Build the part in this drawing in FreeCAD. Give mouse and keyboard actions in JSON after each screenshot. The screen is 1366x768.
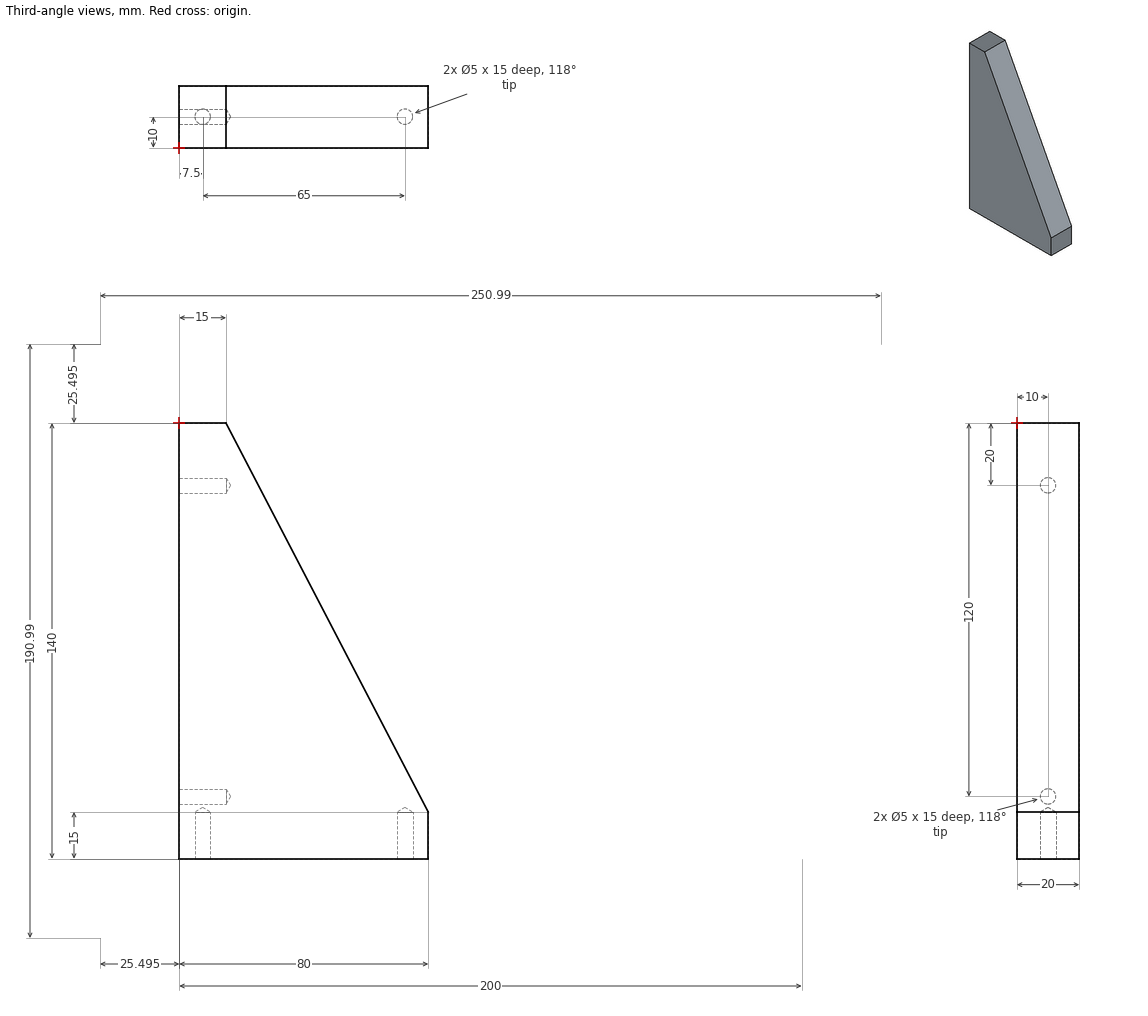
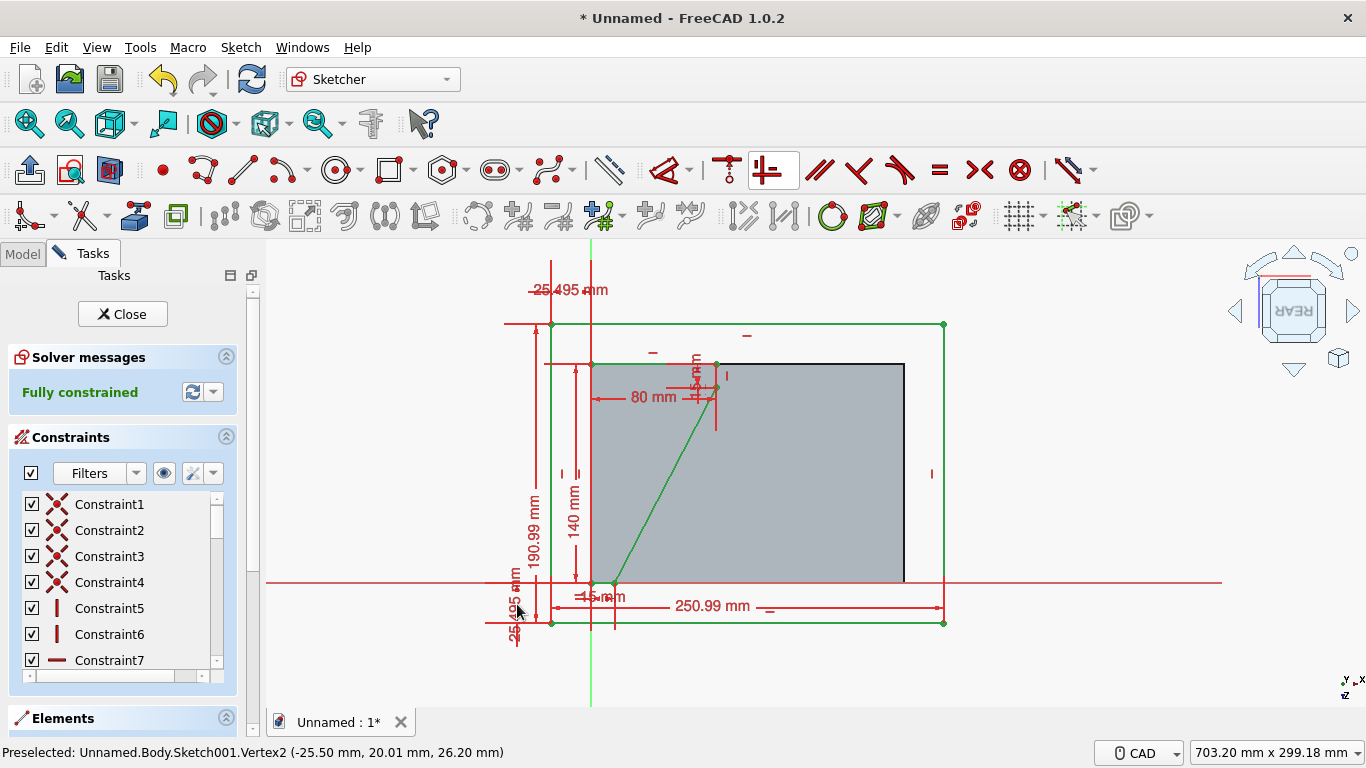
{"action": "left_click", "coordinate": [123, 314]}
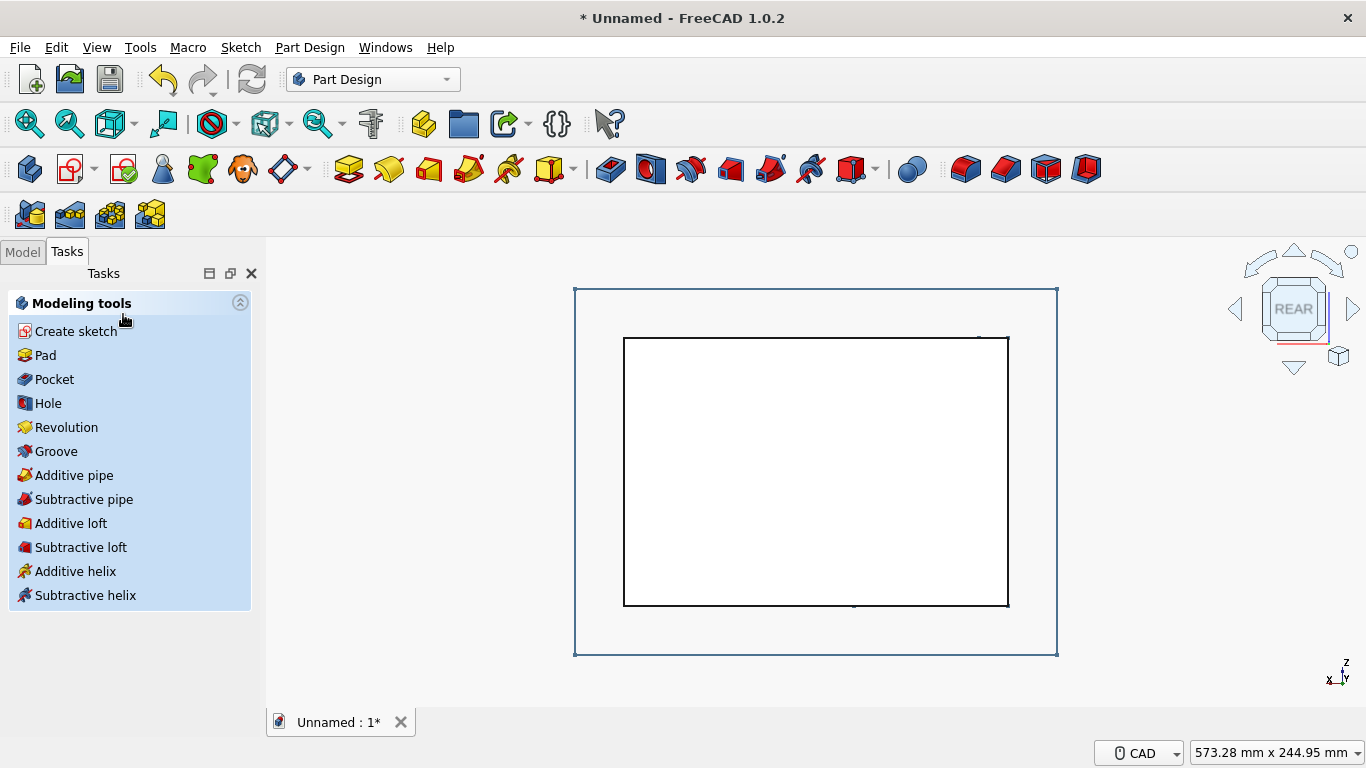
{"action": "left_click", "coordinate": [612, 170]}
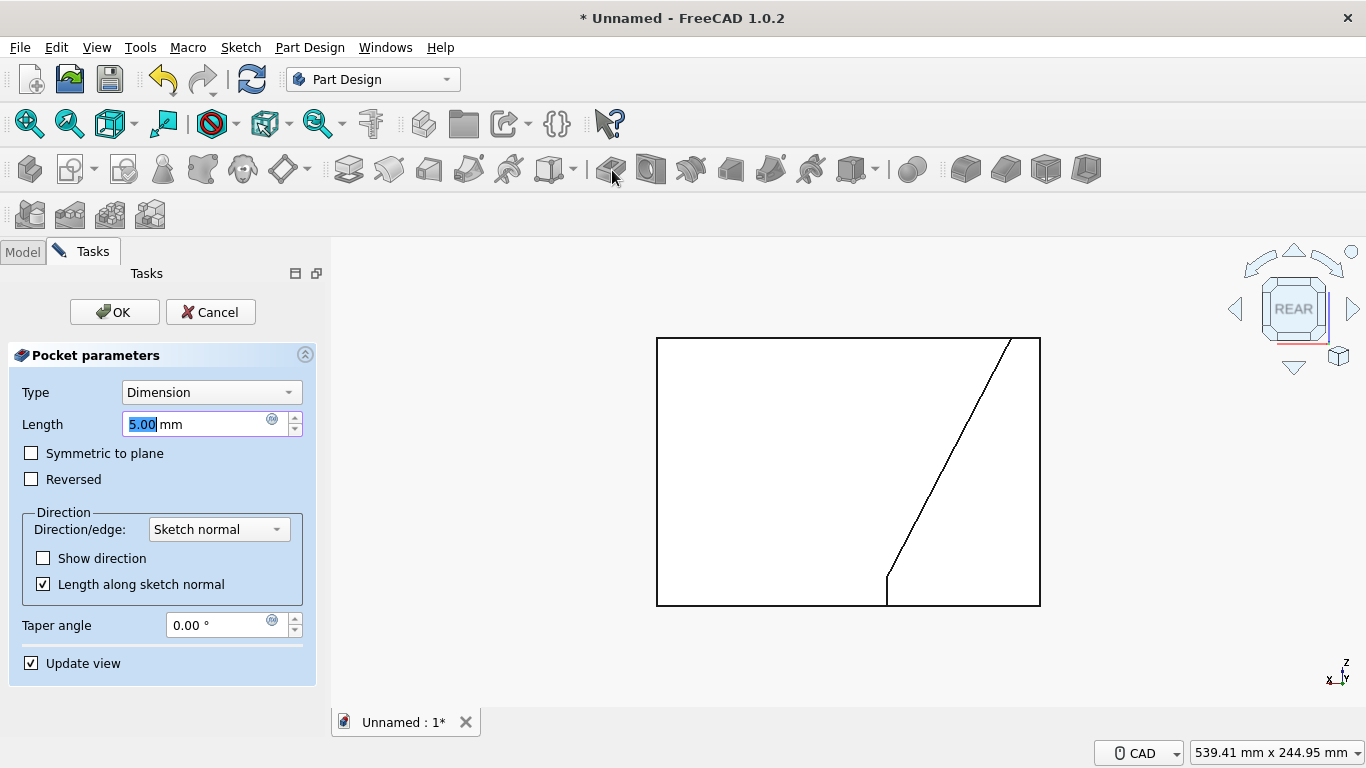
{"action": "left_click", "coordinate": [212, 392]}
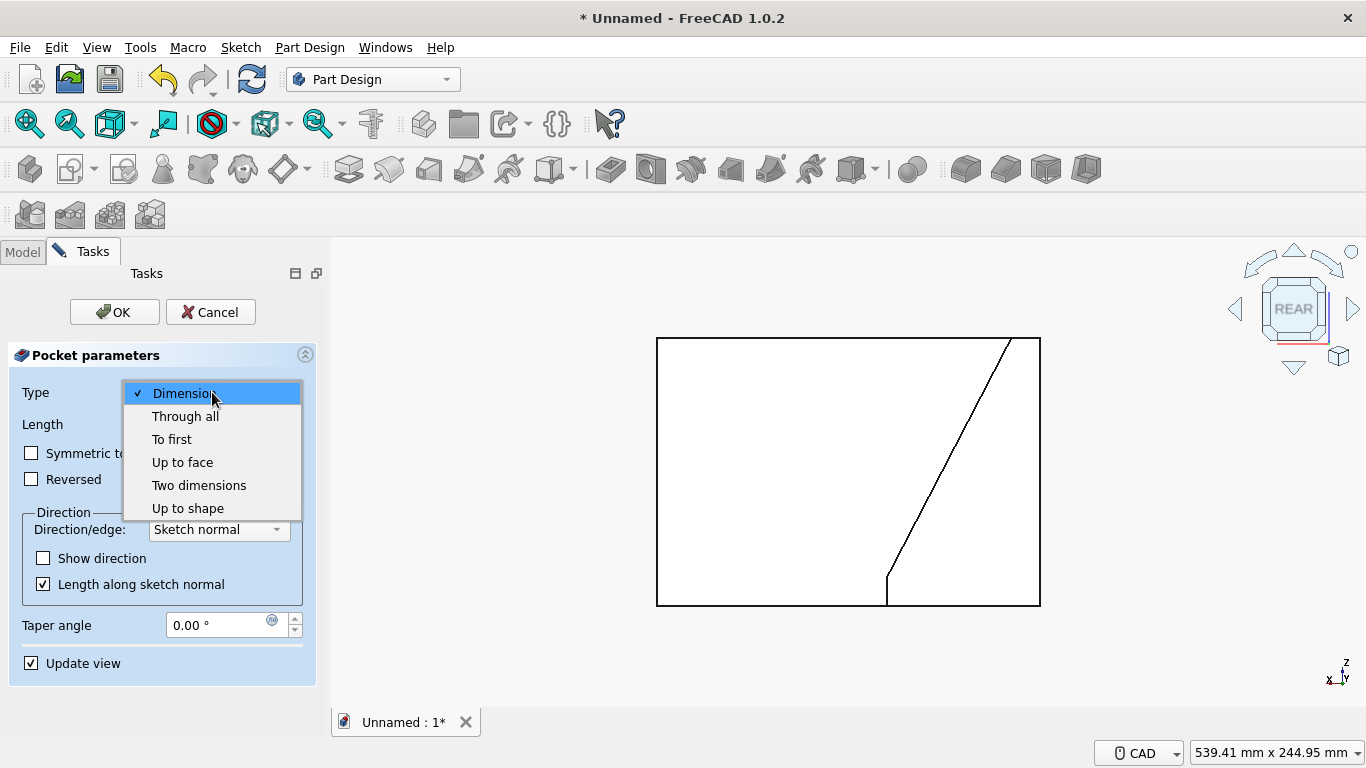
{"action": "left_click", "coordinate": [212, 416]}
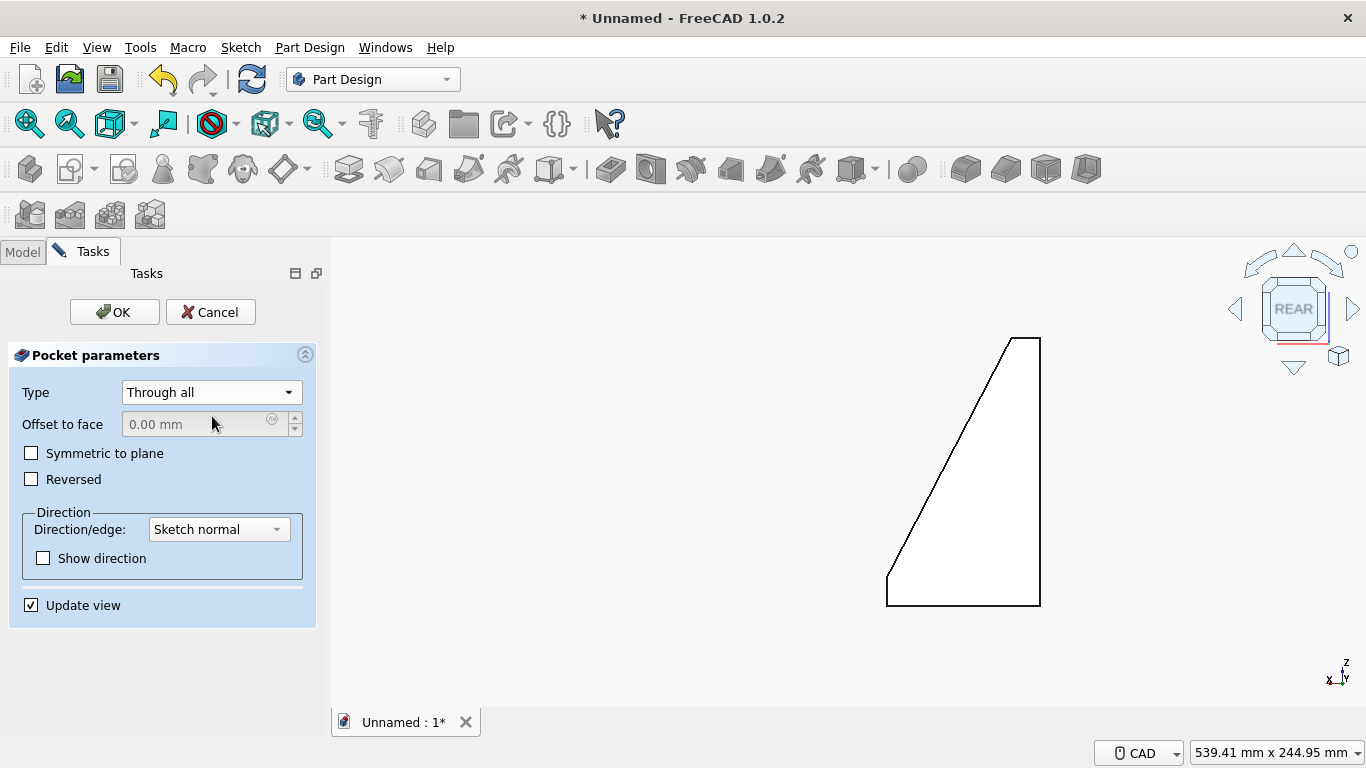
{"action": "left_click", "coordinate": [115, 312]}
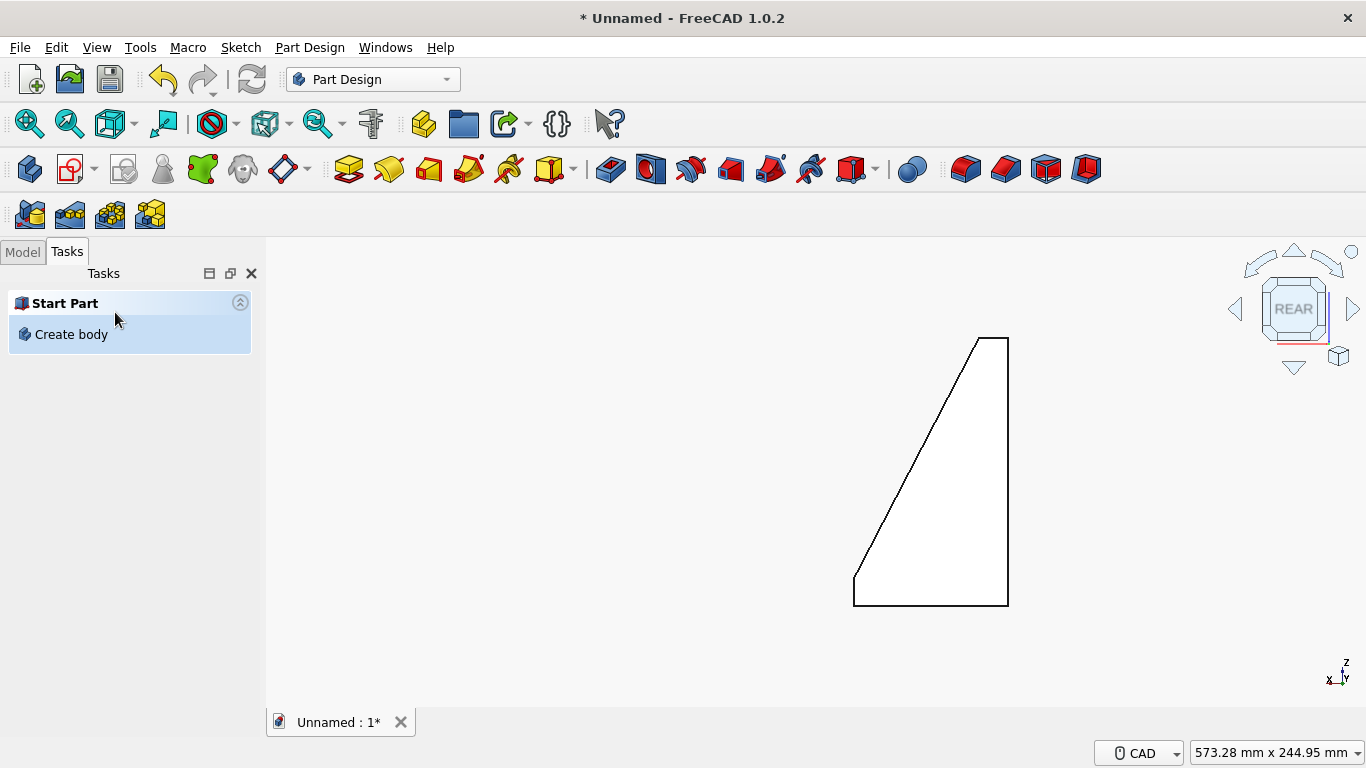
{"action": "left_click", "coordinate": [70, 170]}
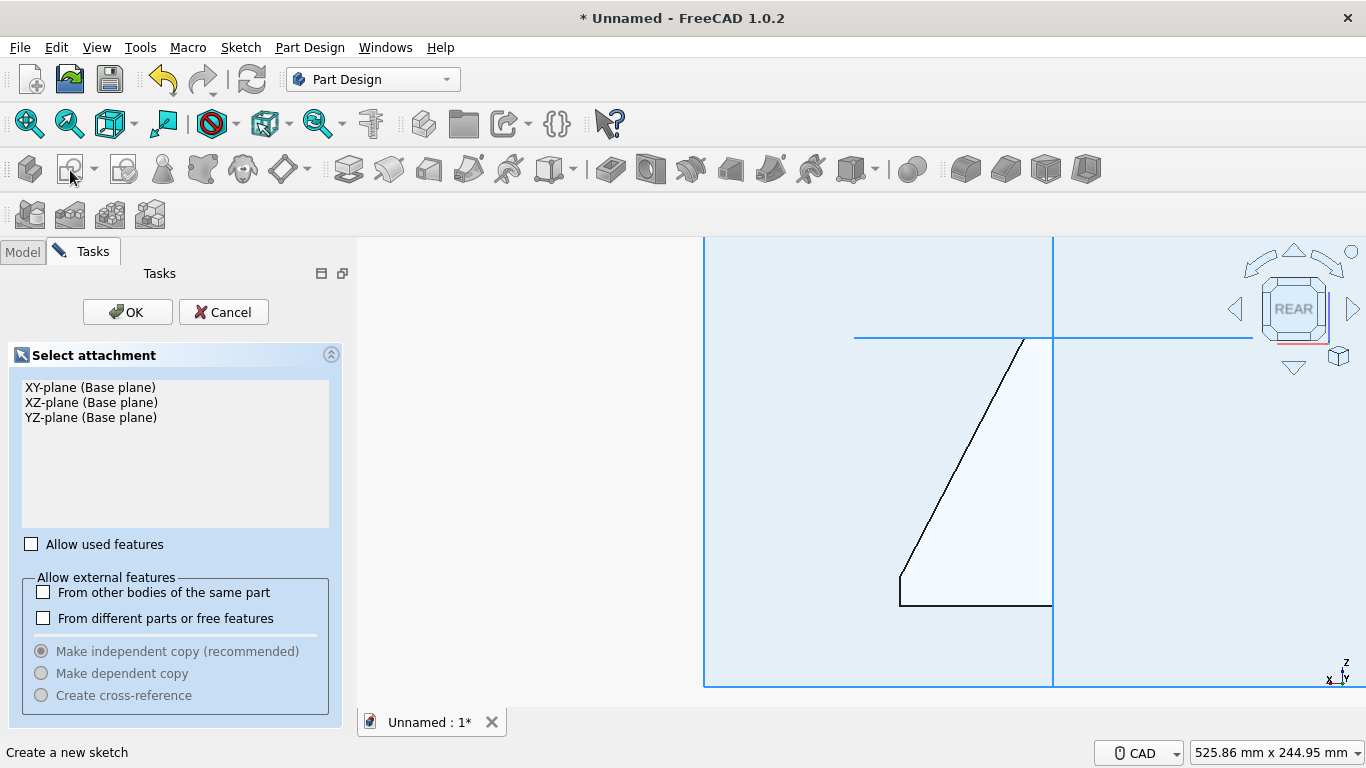
{"action": "left_click", "coordinate": [82, 418]}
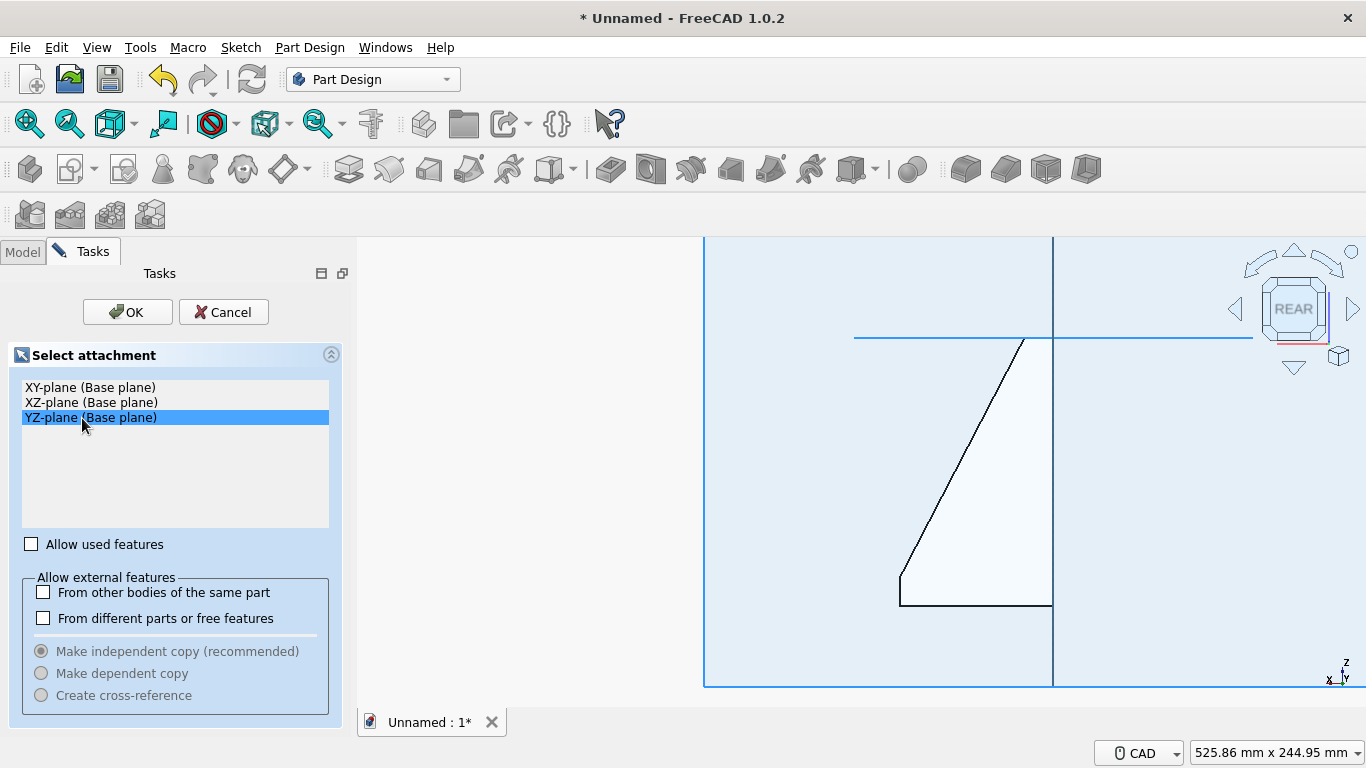
{"action": "left_click", "coordinate": [128, 312]}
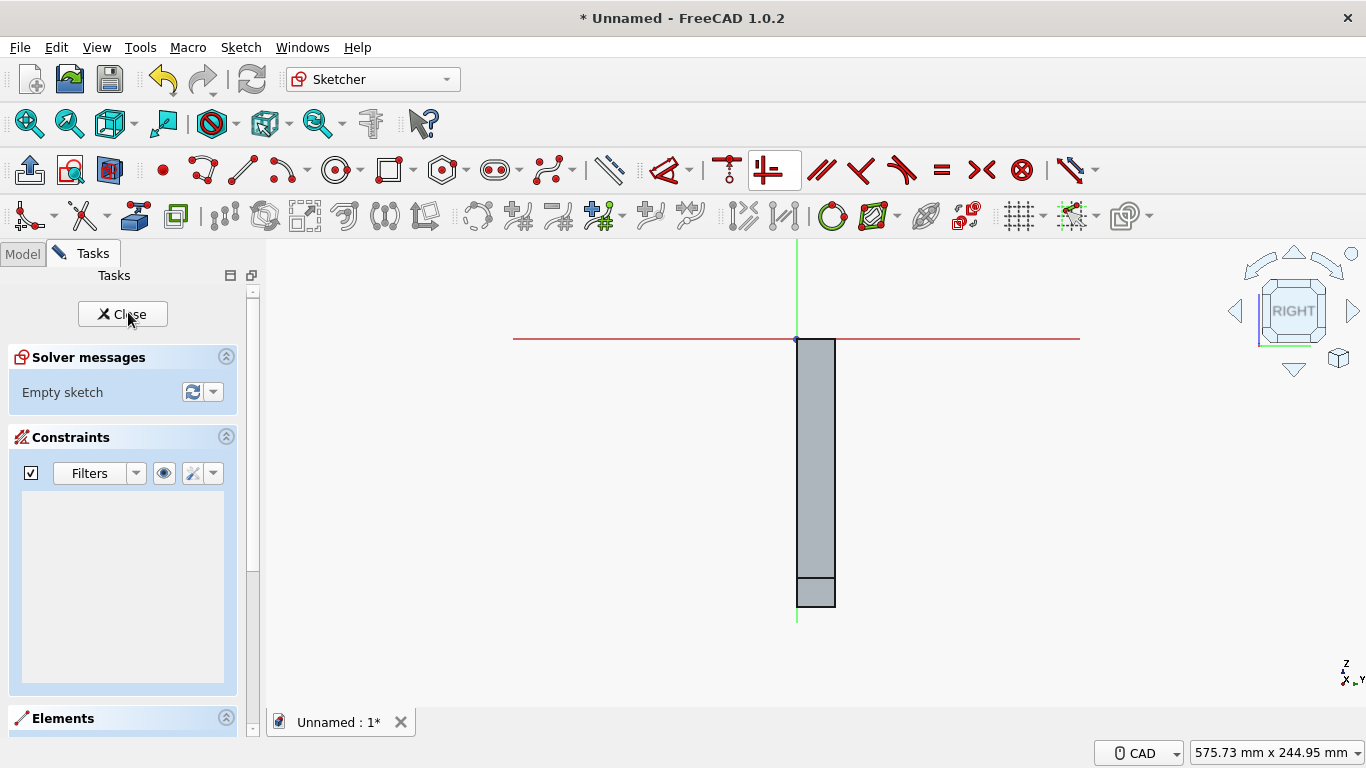
{"action": "left_click", "coordinate": [110, 170]}